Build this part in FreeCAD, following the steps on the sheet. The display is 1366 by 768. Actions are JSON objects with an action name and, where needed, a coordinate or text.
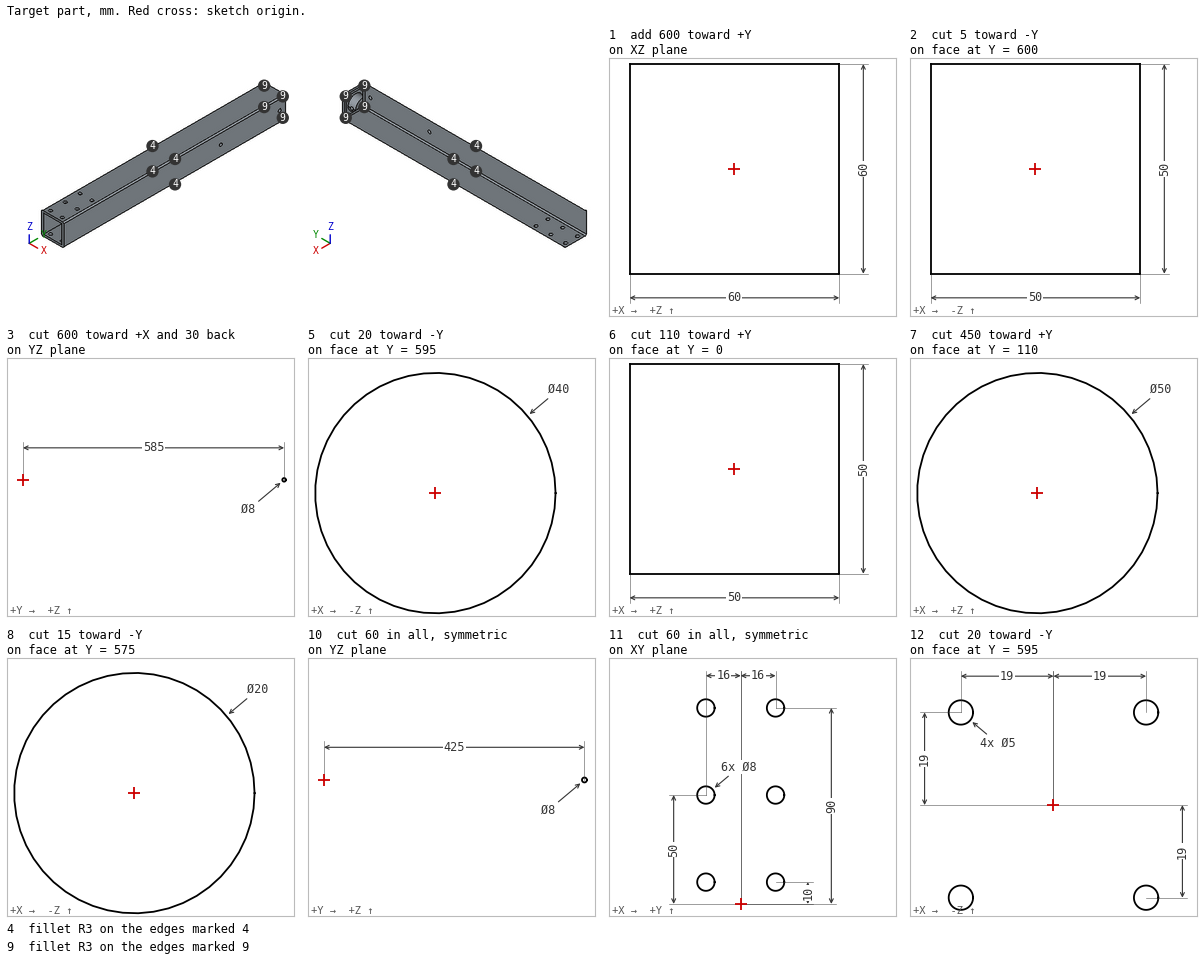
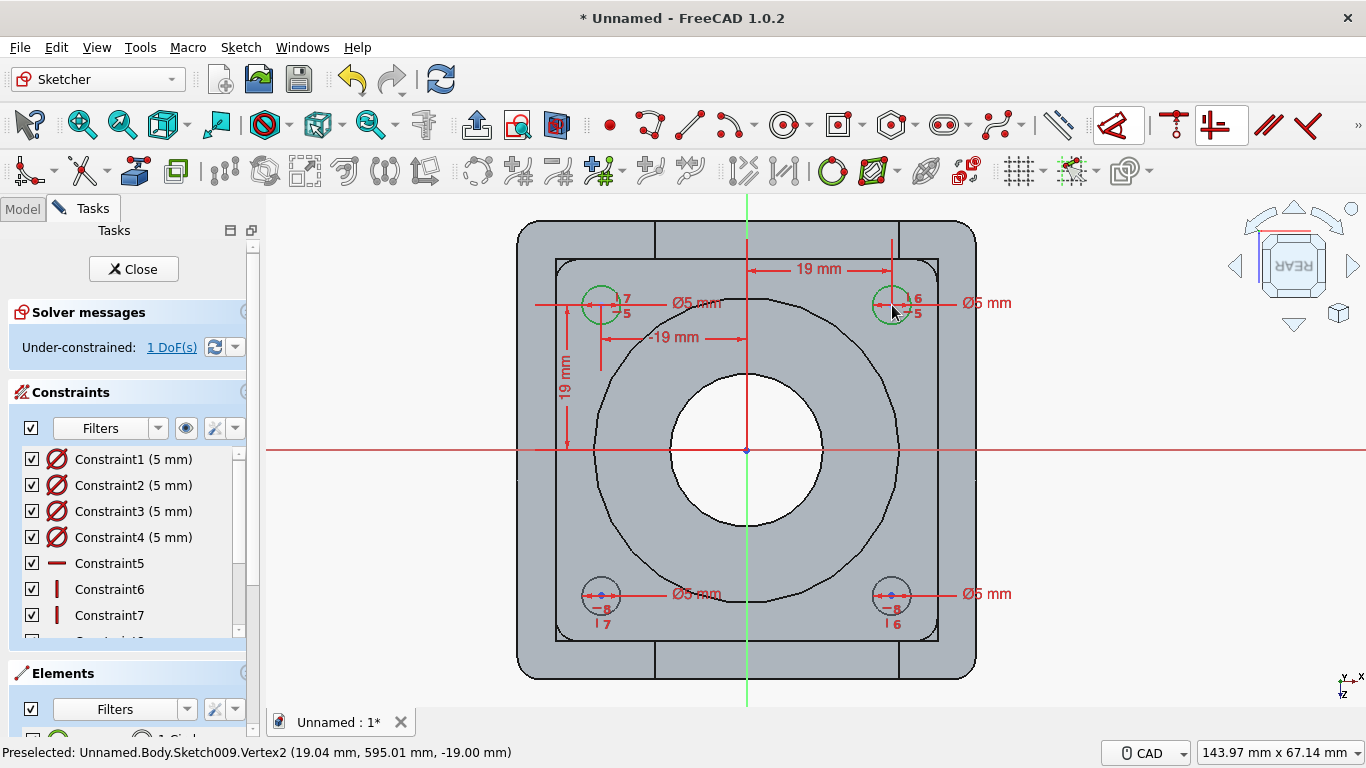
{"action": "left_click", "coordinate": [892, 596]}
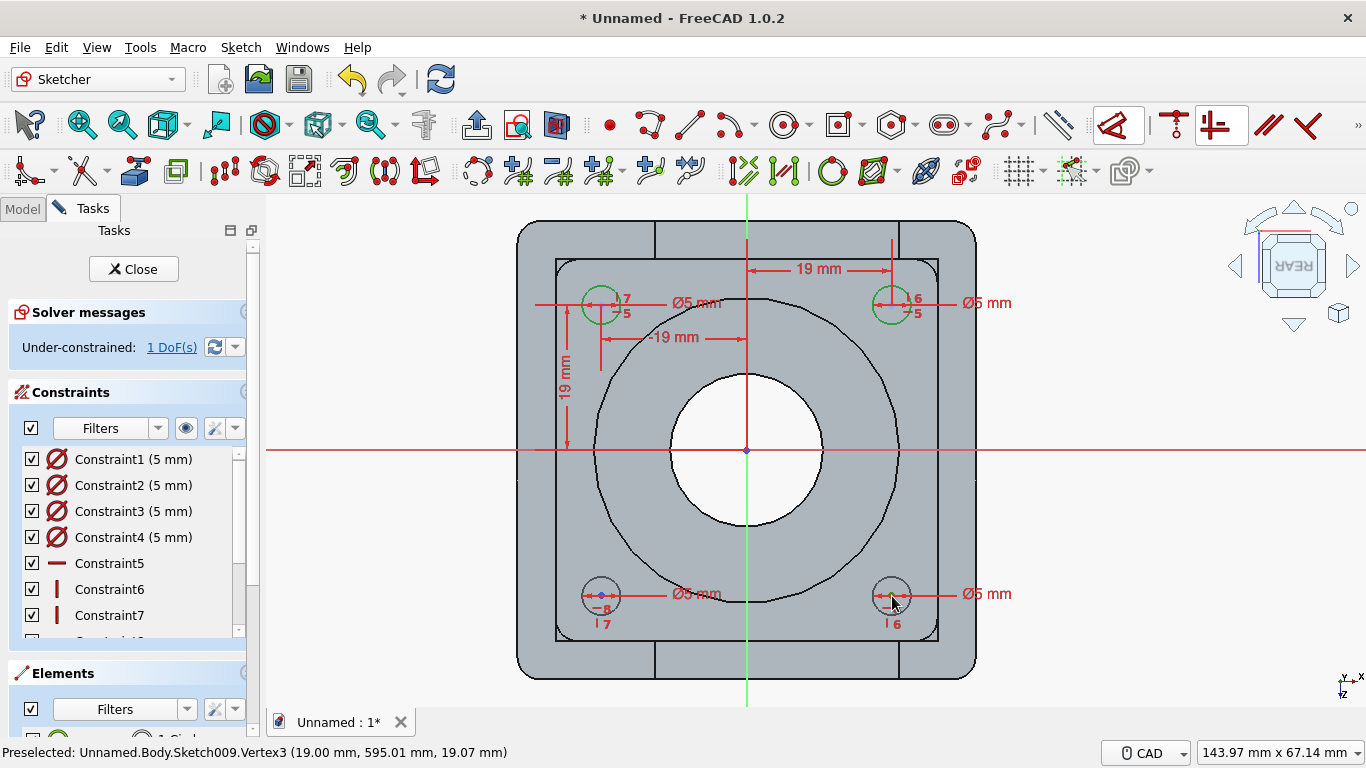
{"action": "left_click", "coordinate": [1138, 126]}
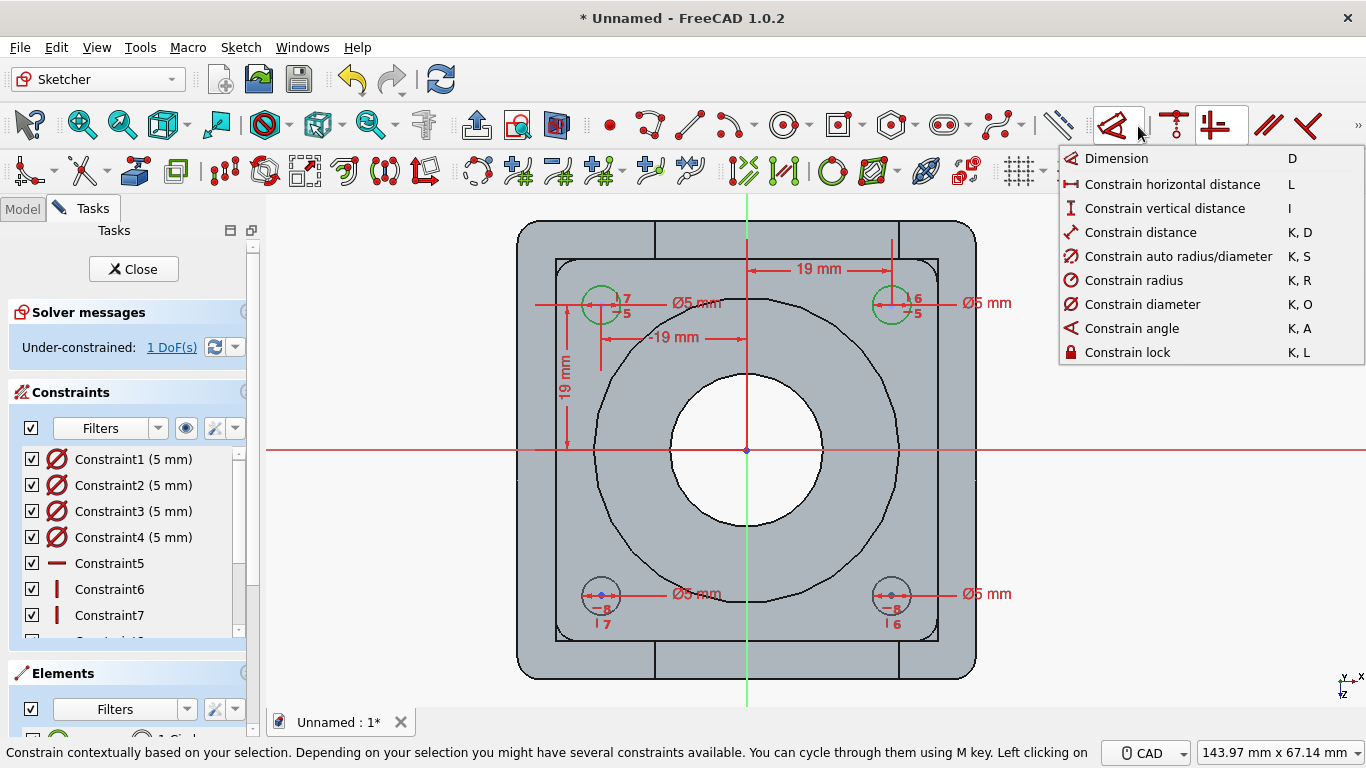
{"action": "left_click", "coordinate": [1212, 208]}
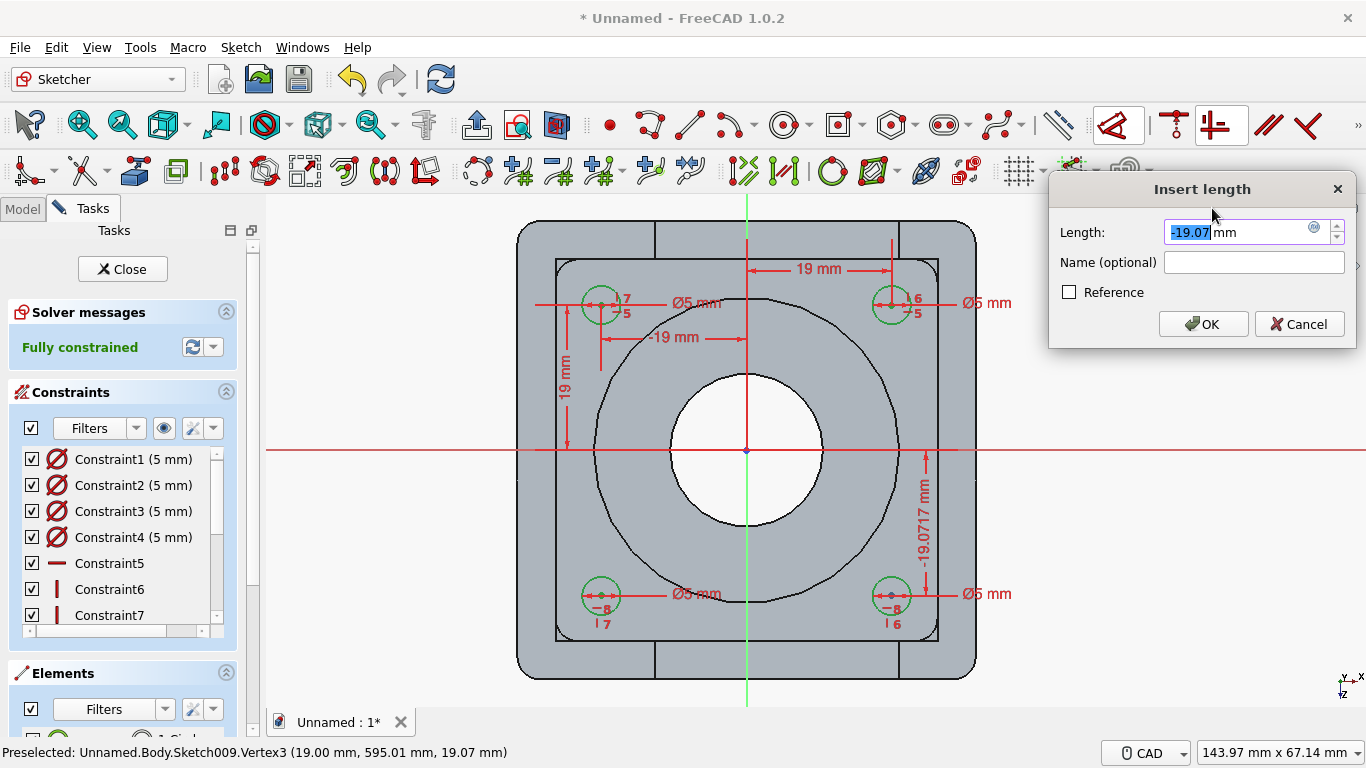
{"action": "type", "text": "-19"}
{"action": "key", "text": "Return"}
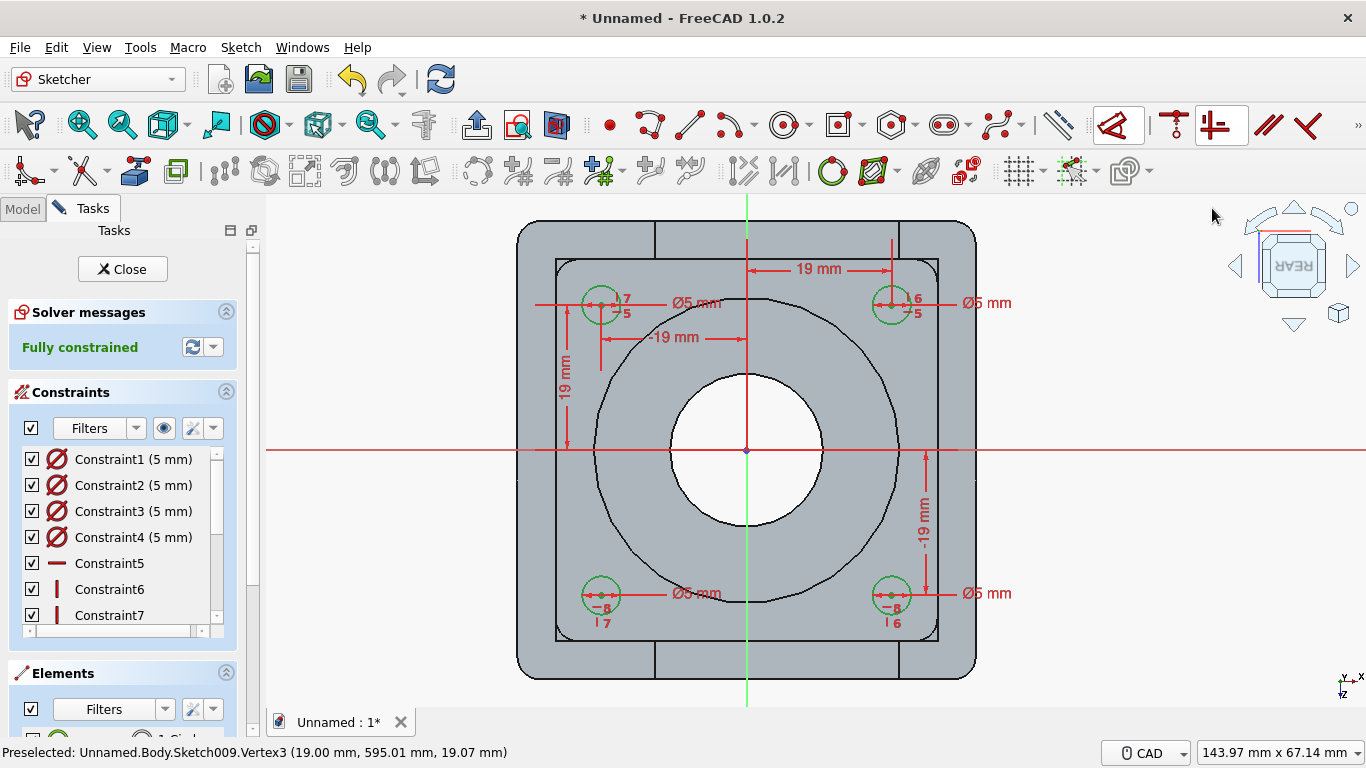
{"action": "left_click", "coordinate": [123, 269]}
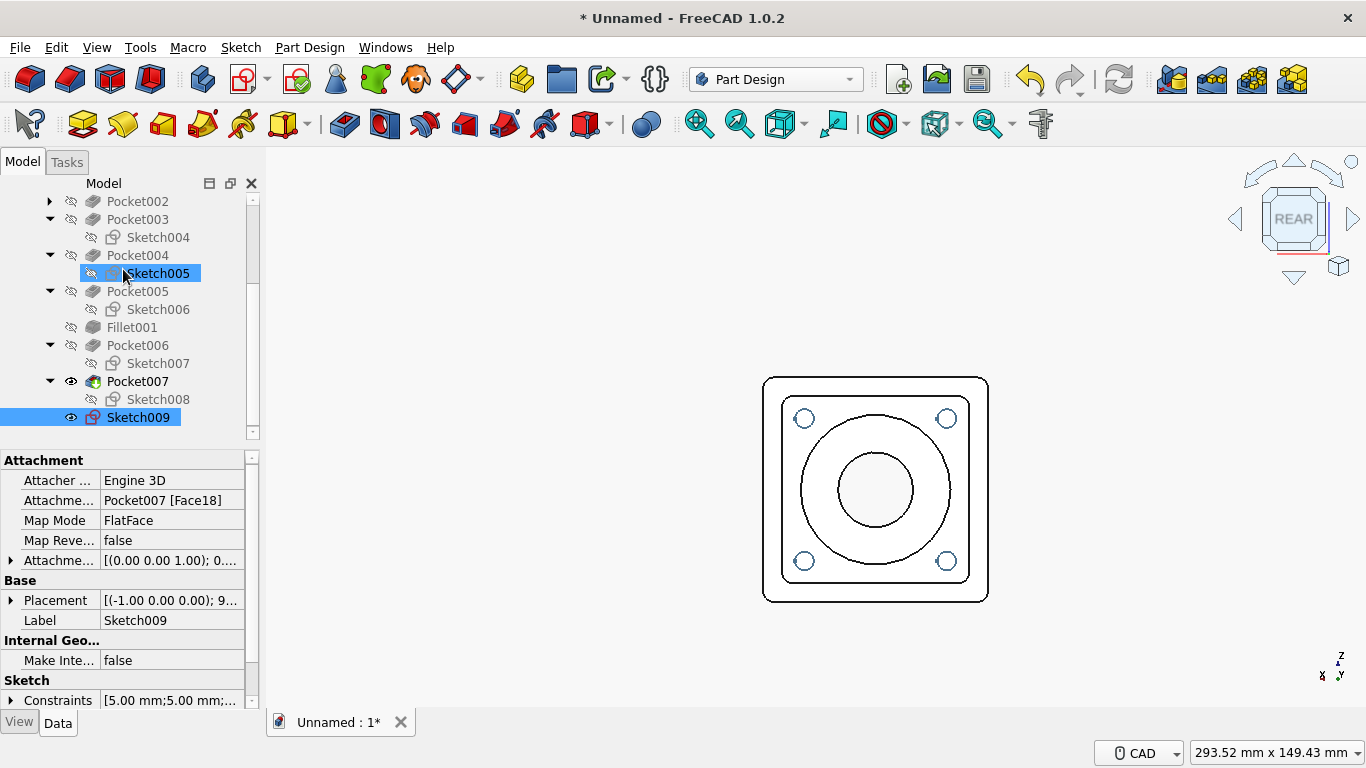
{"action": "left_click", "coordinate": [346, 124]}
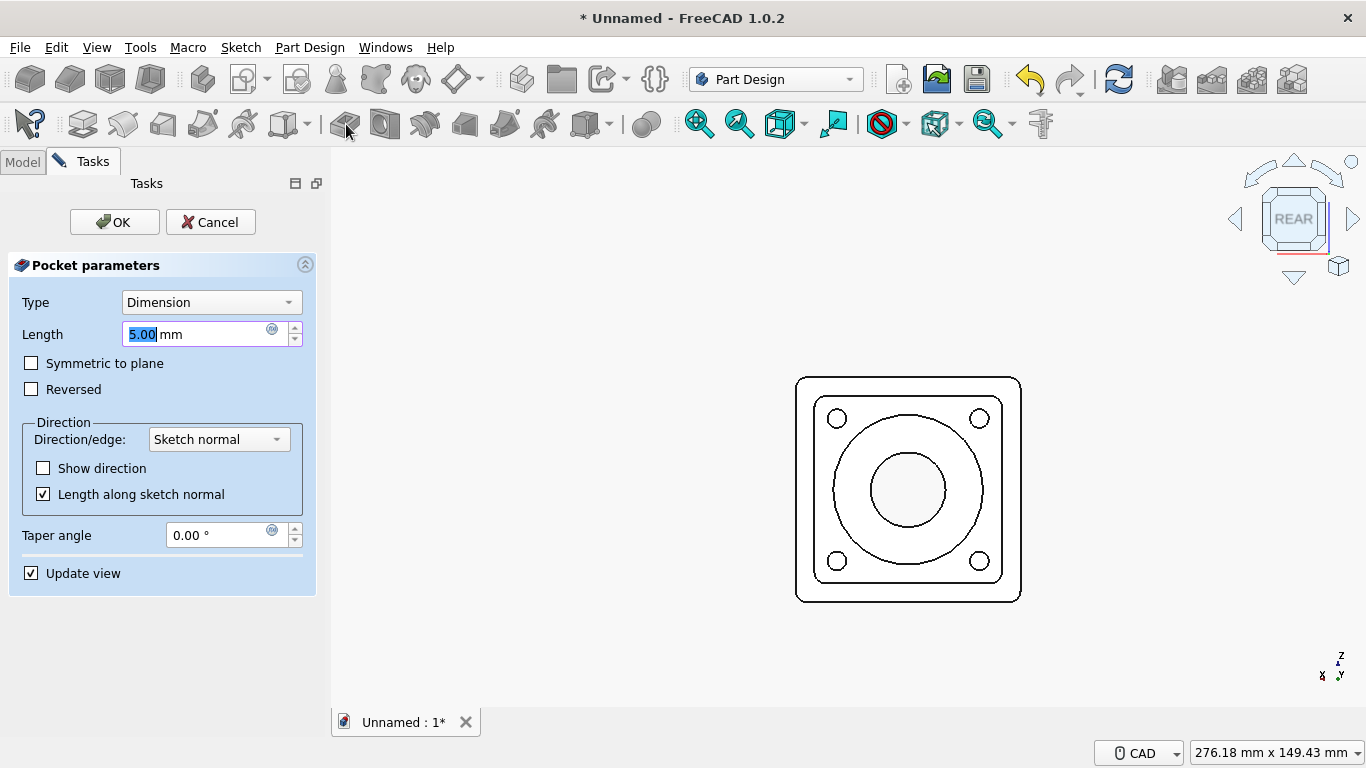
{"action": "type", "text": "20"}
{"action": "key", "text": "Tab"}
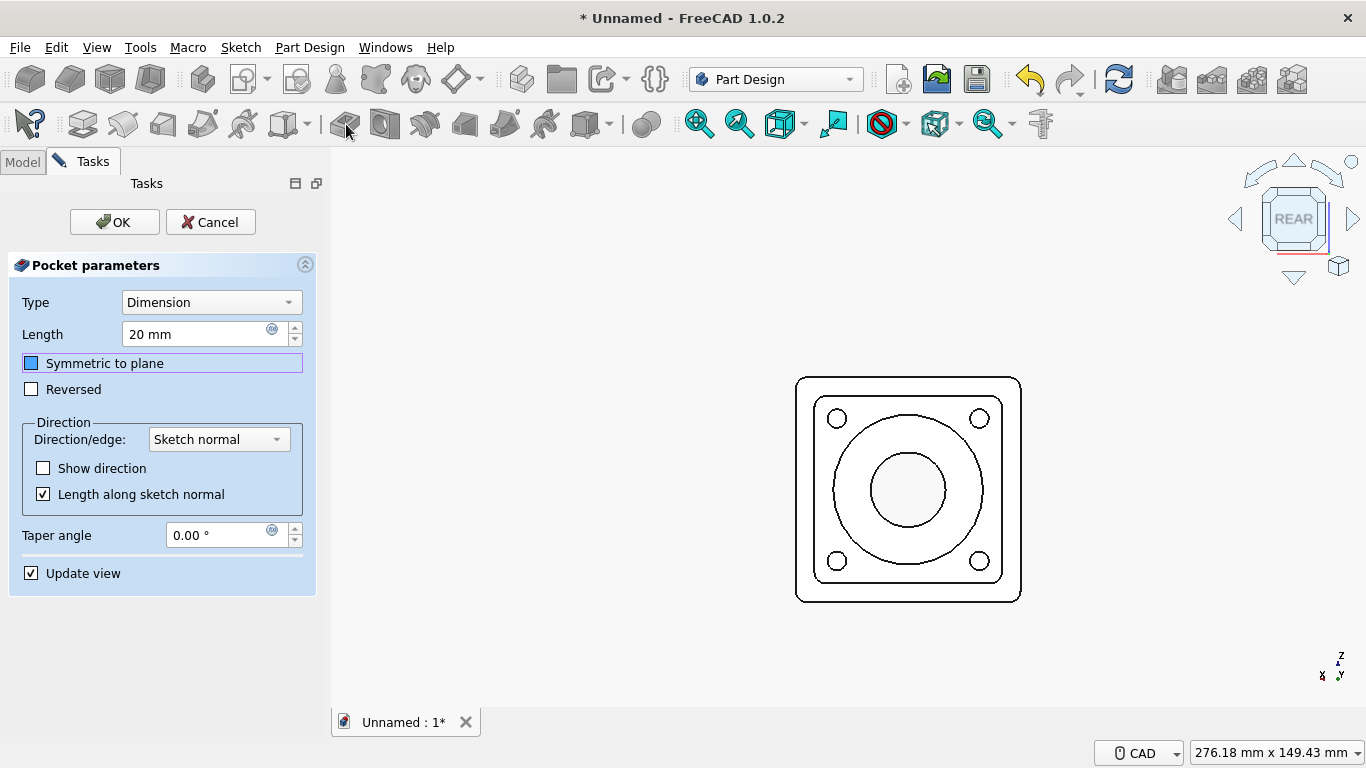
{"action": "left_click", "coordinate": [115, 222]}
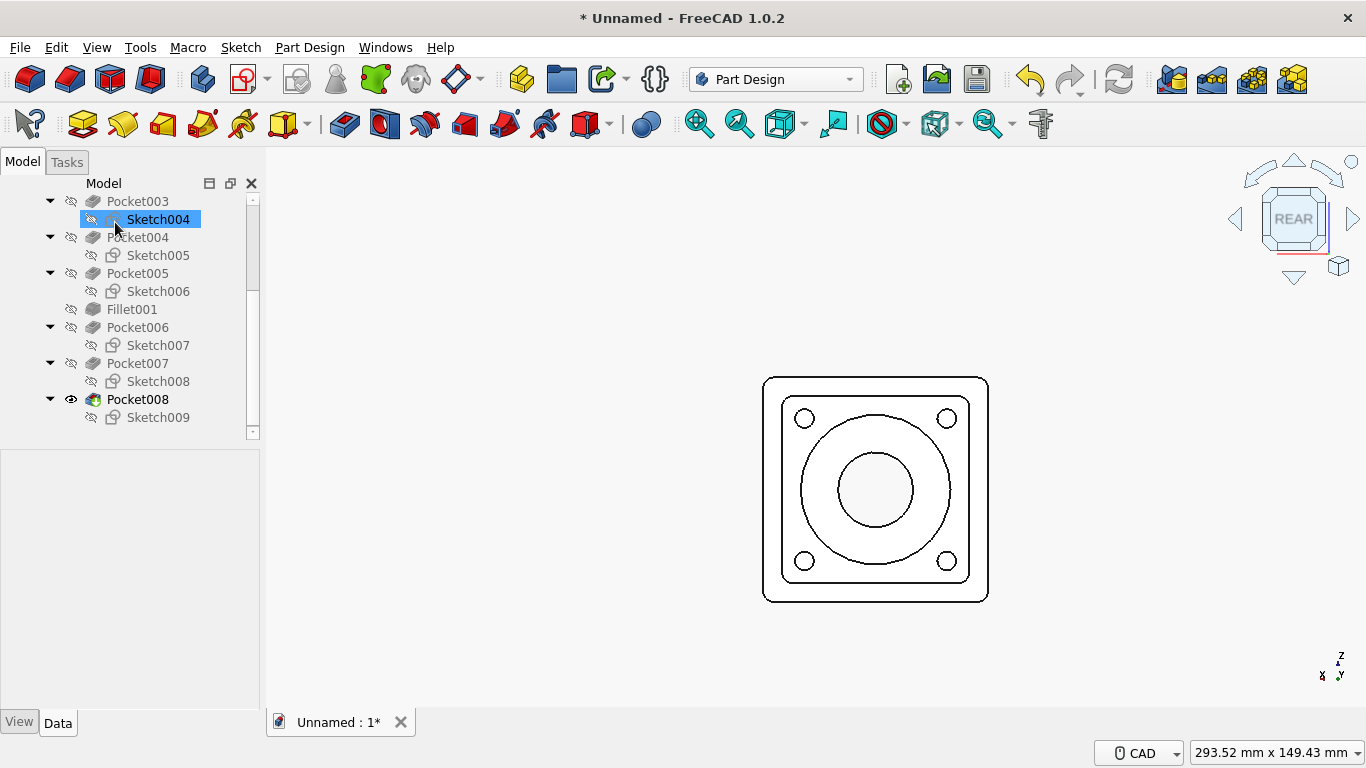
{"action": "key", "text": "0"}